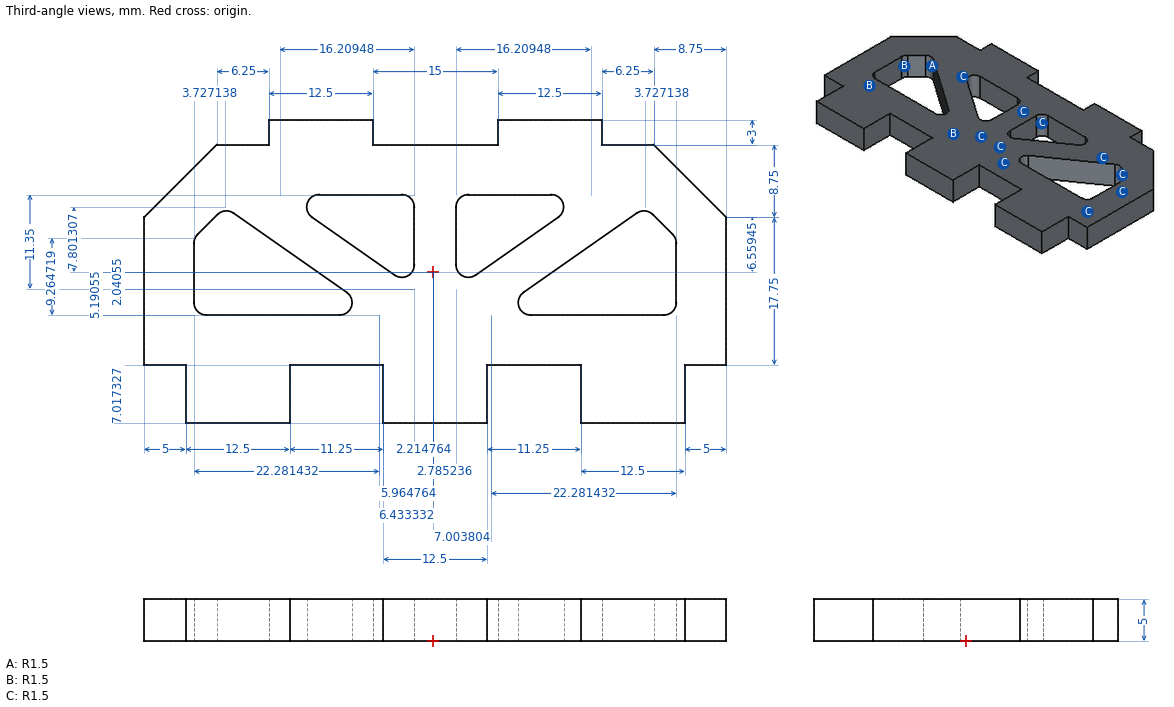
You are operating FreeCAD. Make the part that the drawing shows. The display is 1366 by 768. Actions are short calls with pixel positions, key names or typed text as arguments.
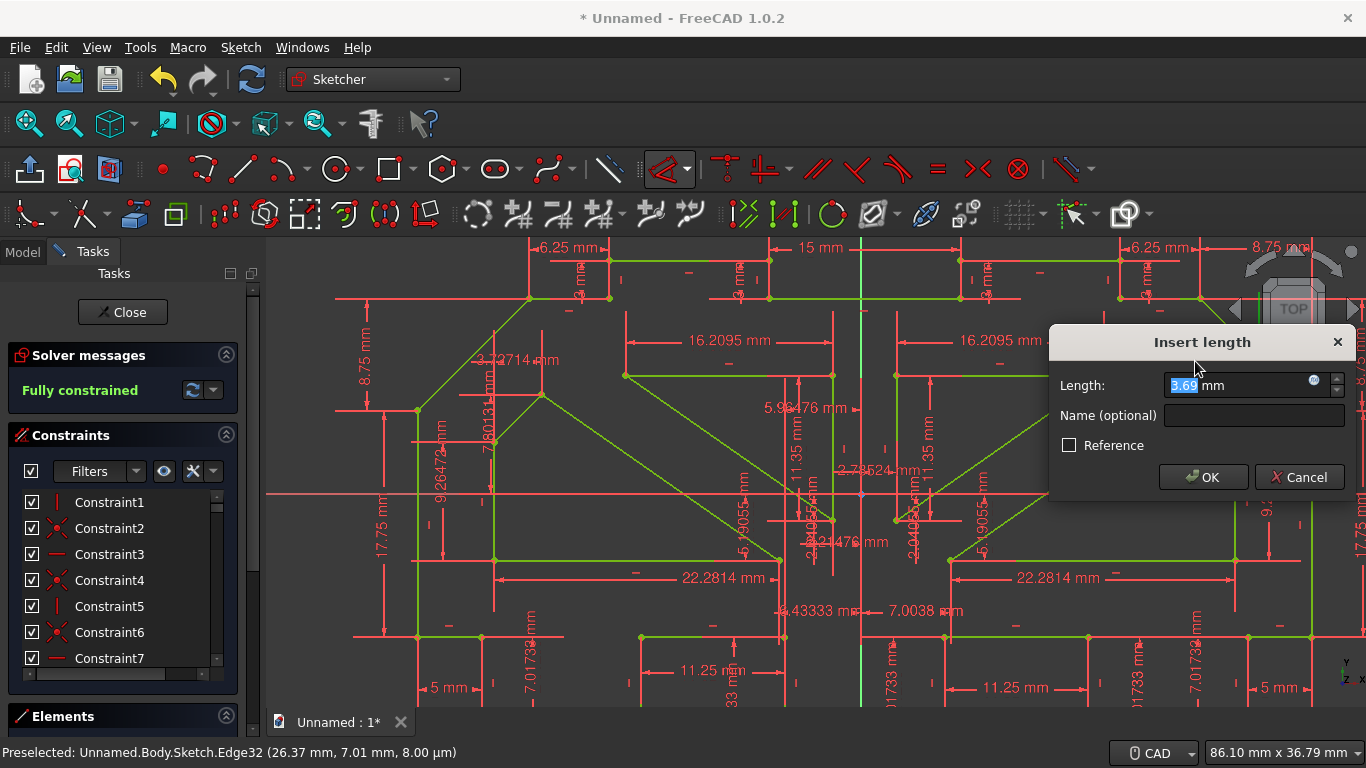
text(3.727138)
key(Return)
key(Escape)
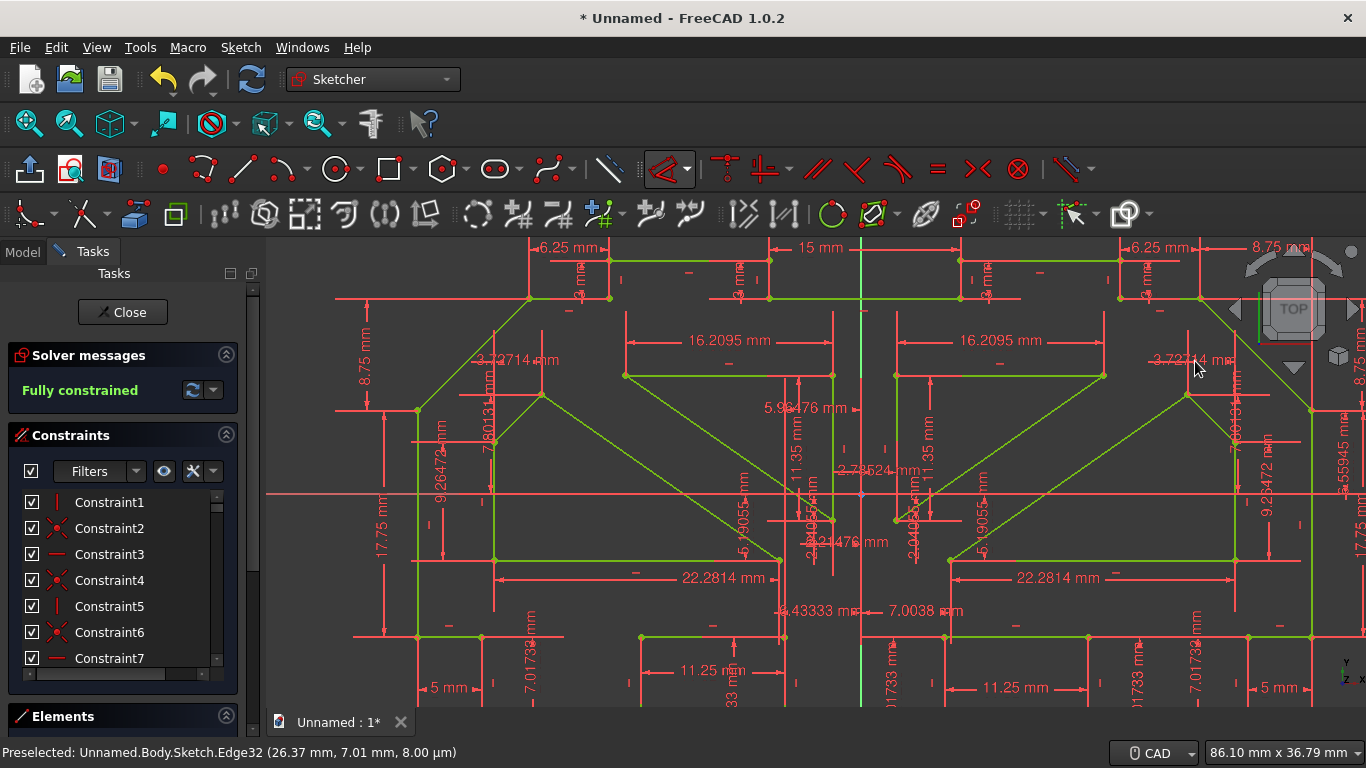
click(123, 312)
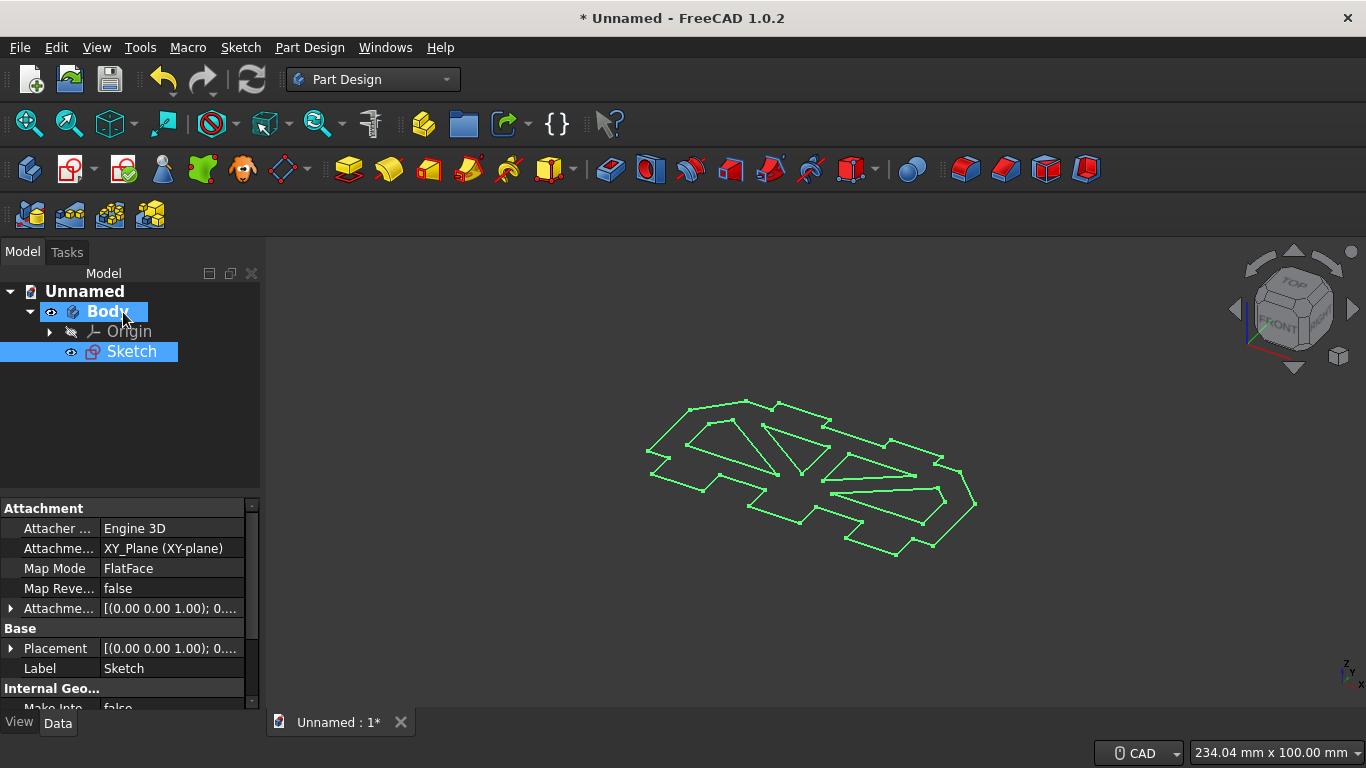
click(350, 170)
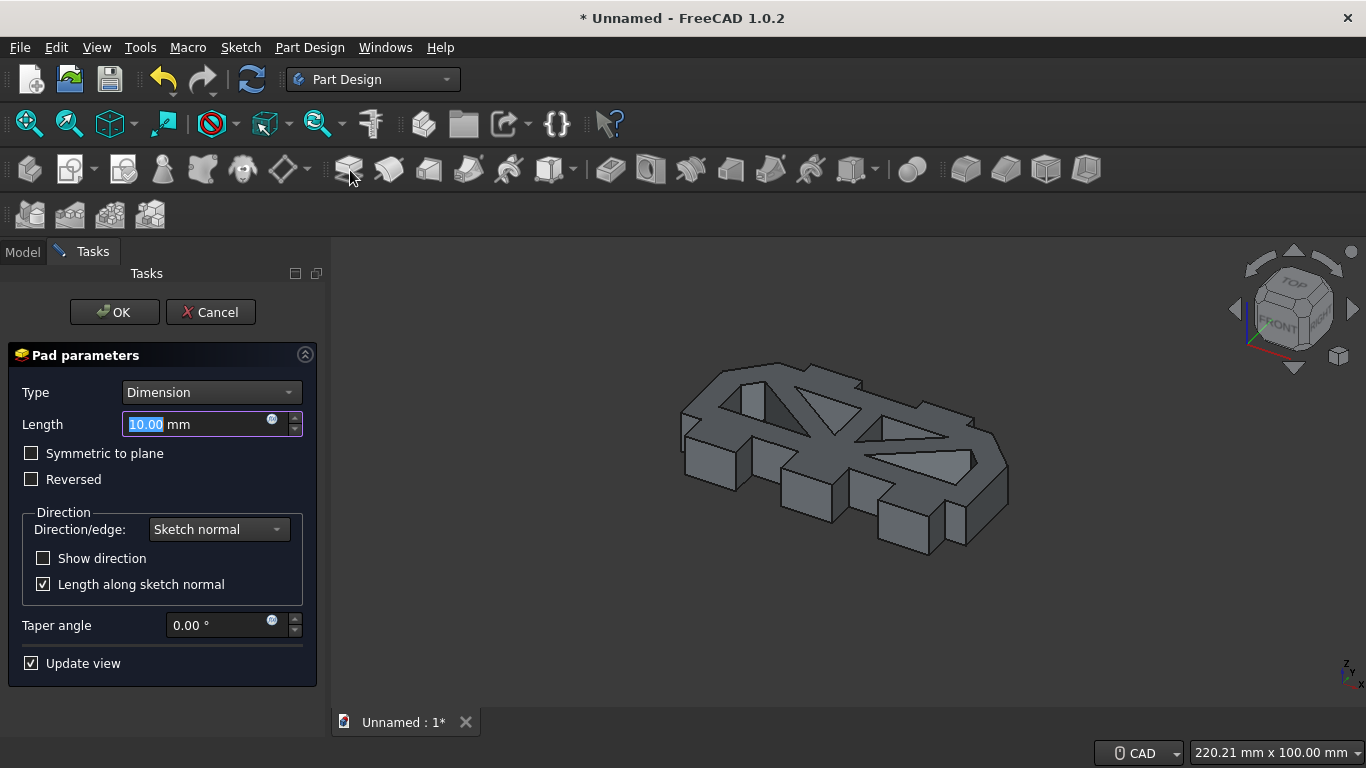
text(5)
key(Tab)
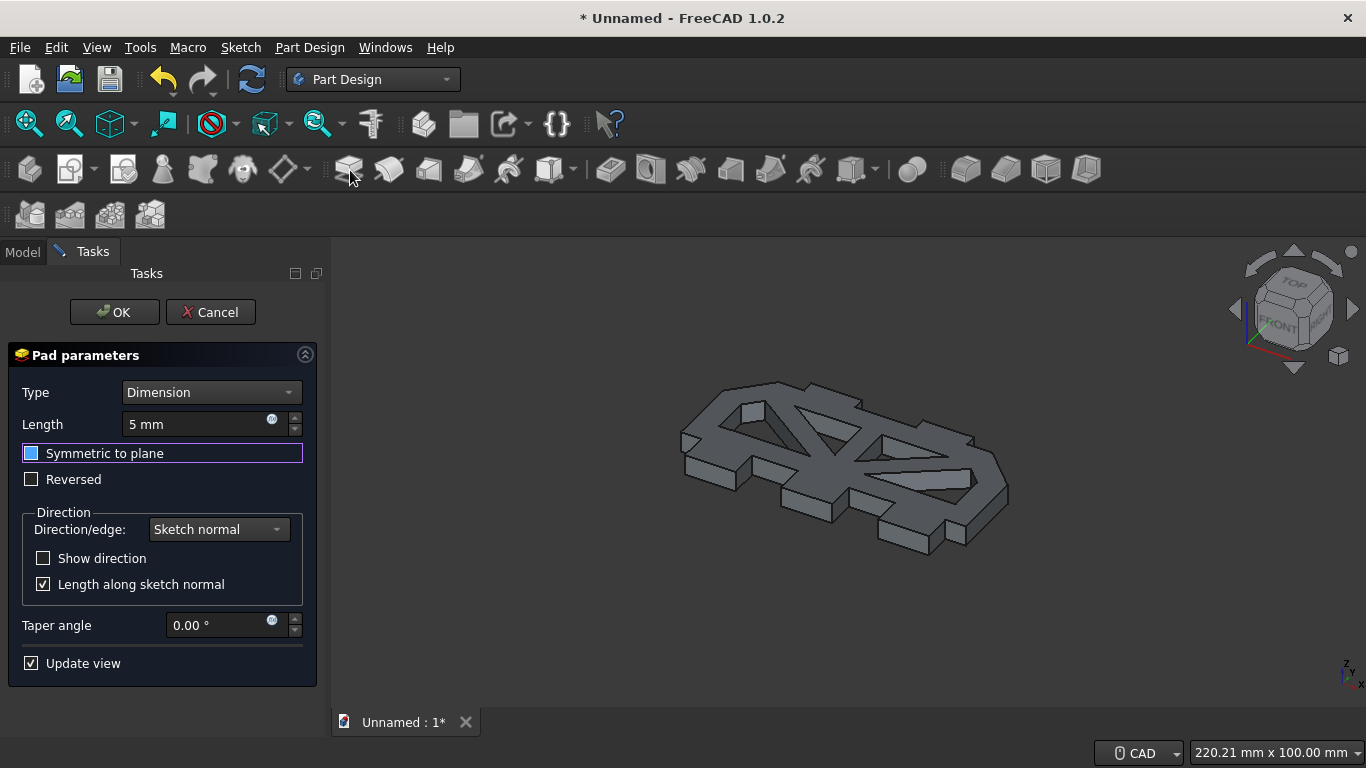
click(115, 312)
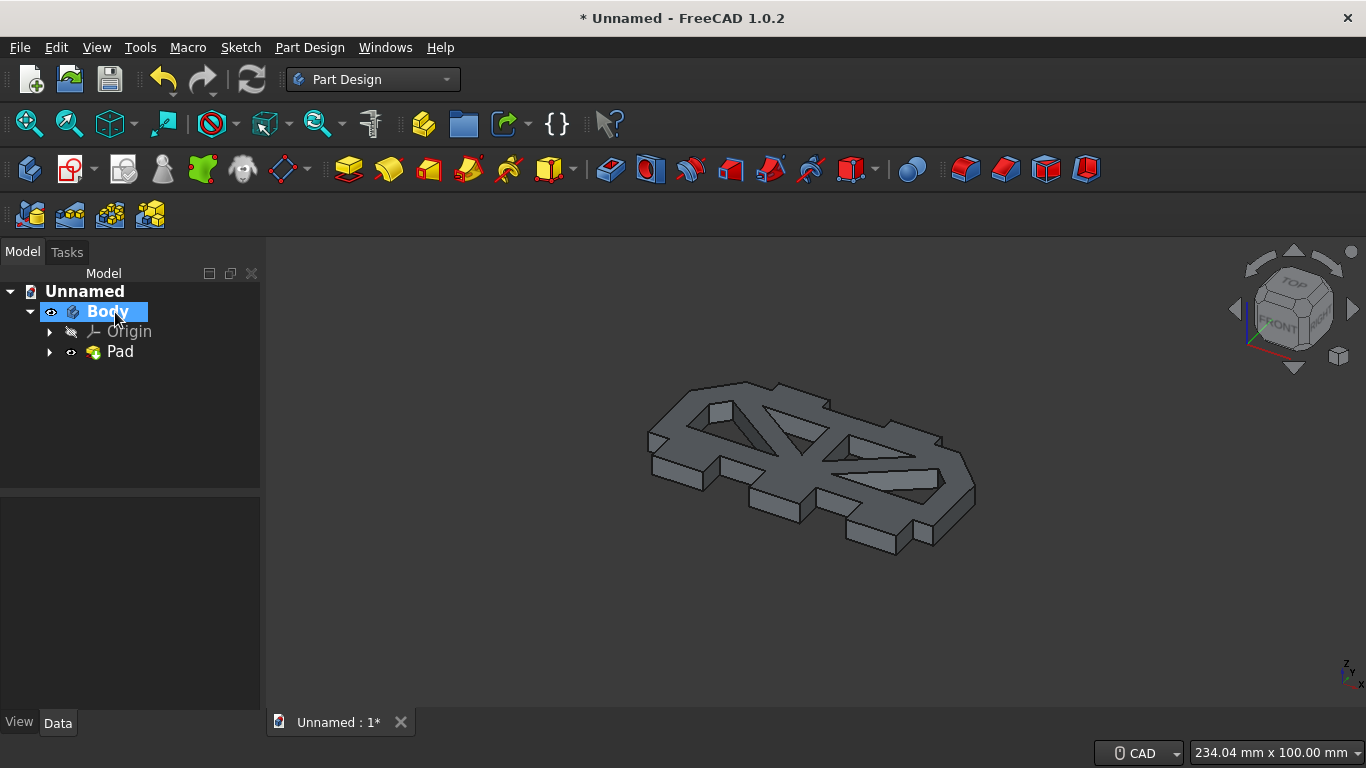
key(v)
key(f)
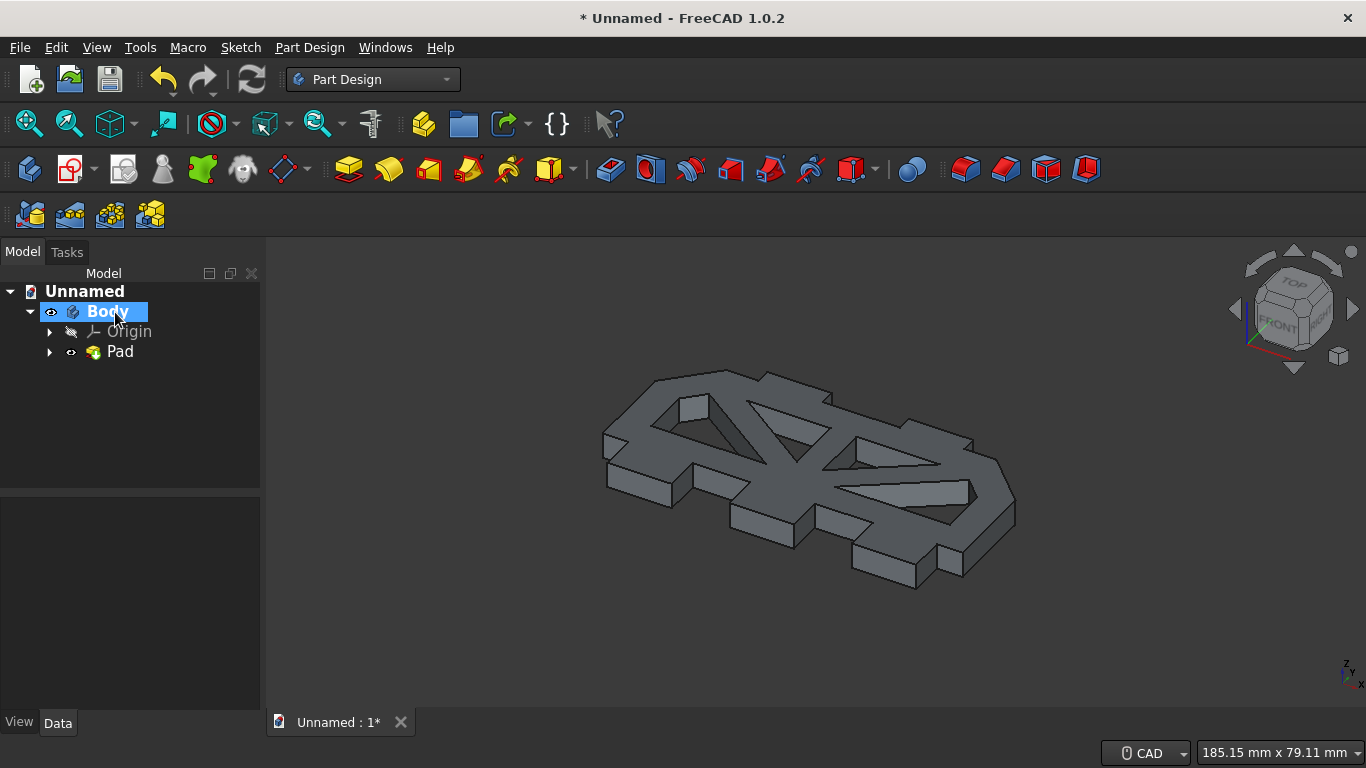
key(0)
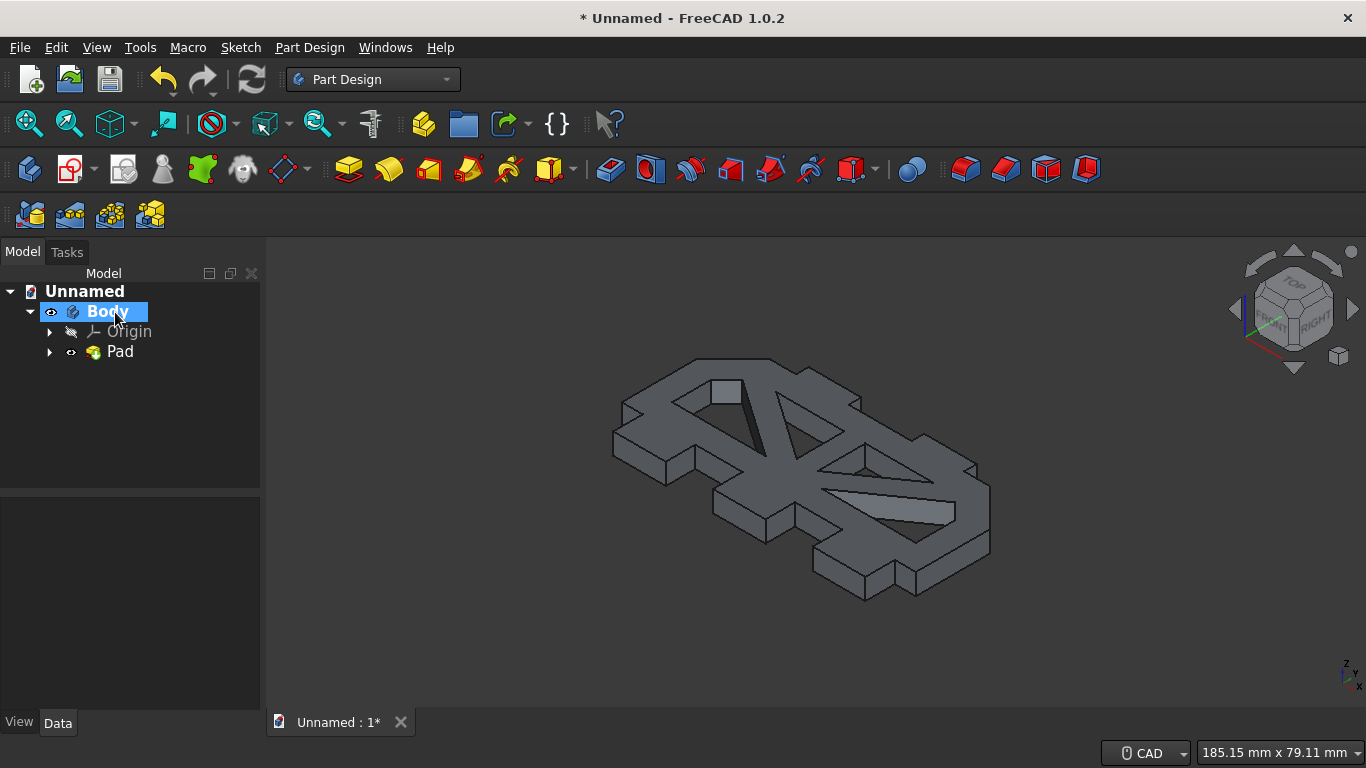
key(2)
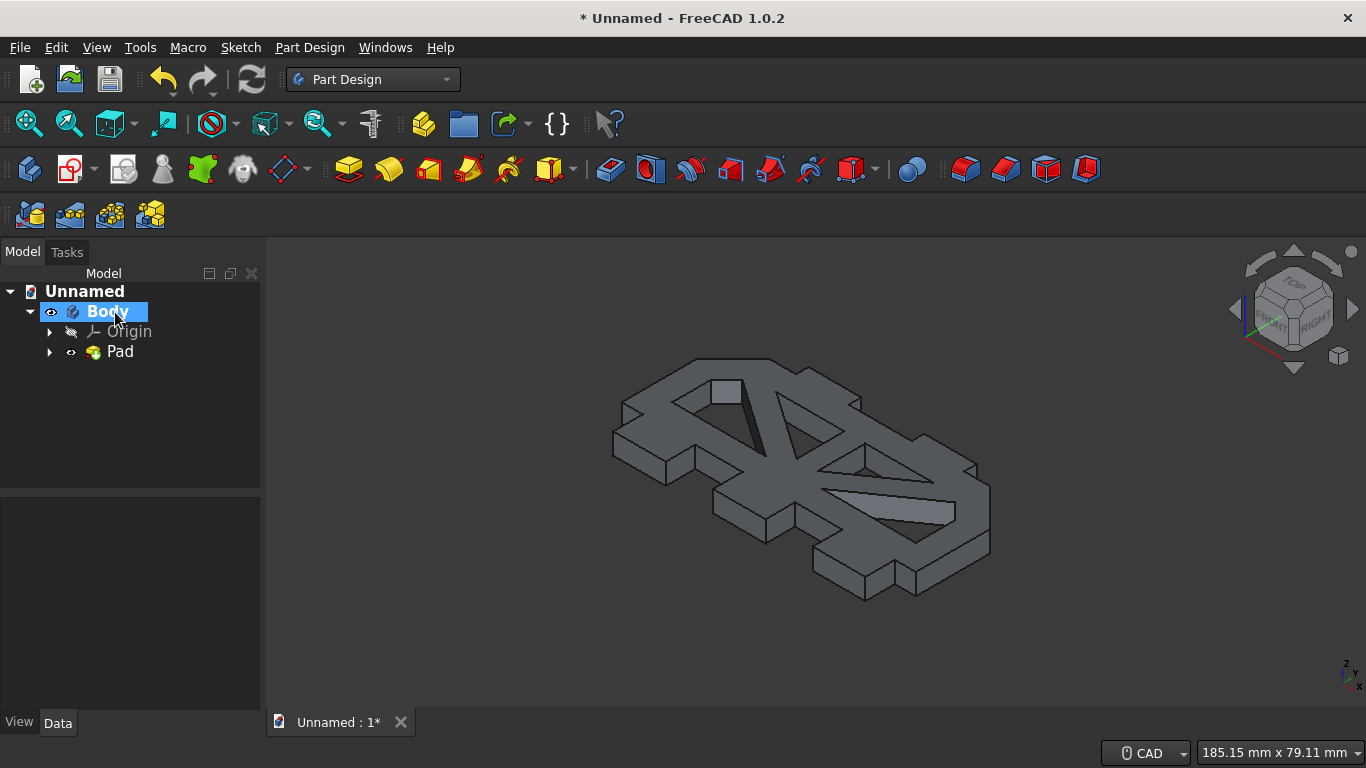
key(1)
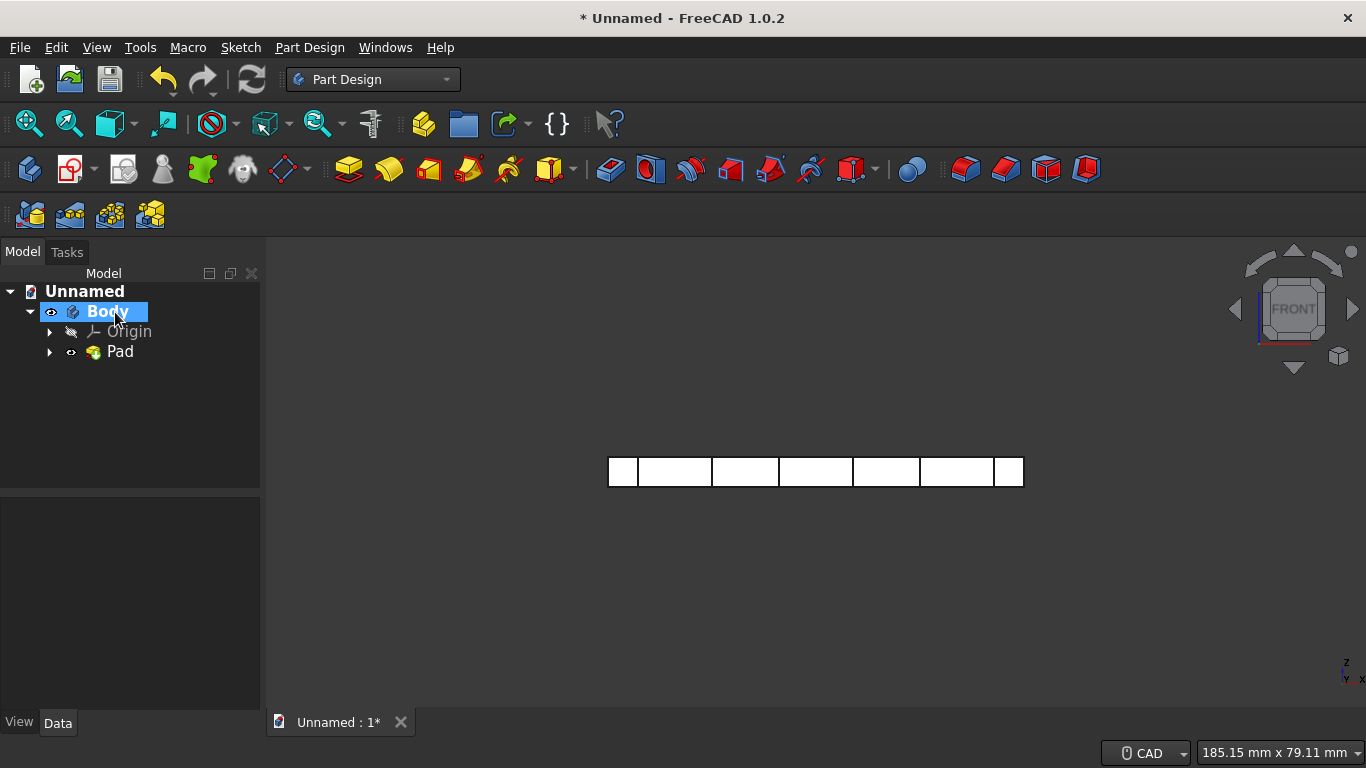
key(v)
key(f)